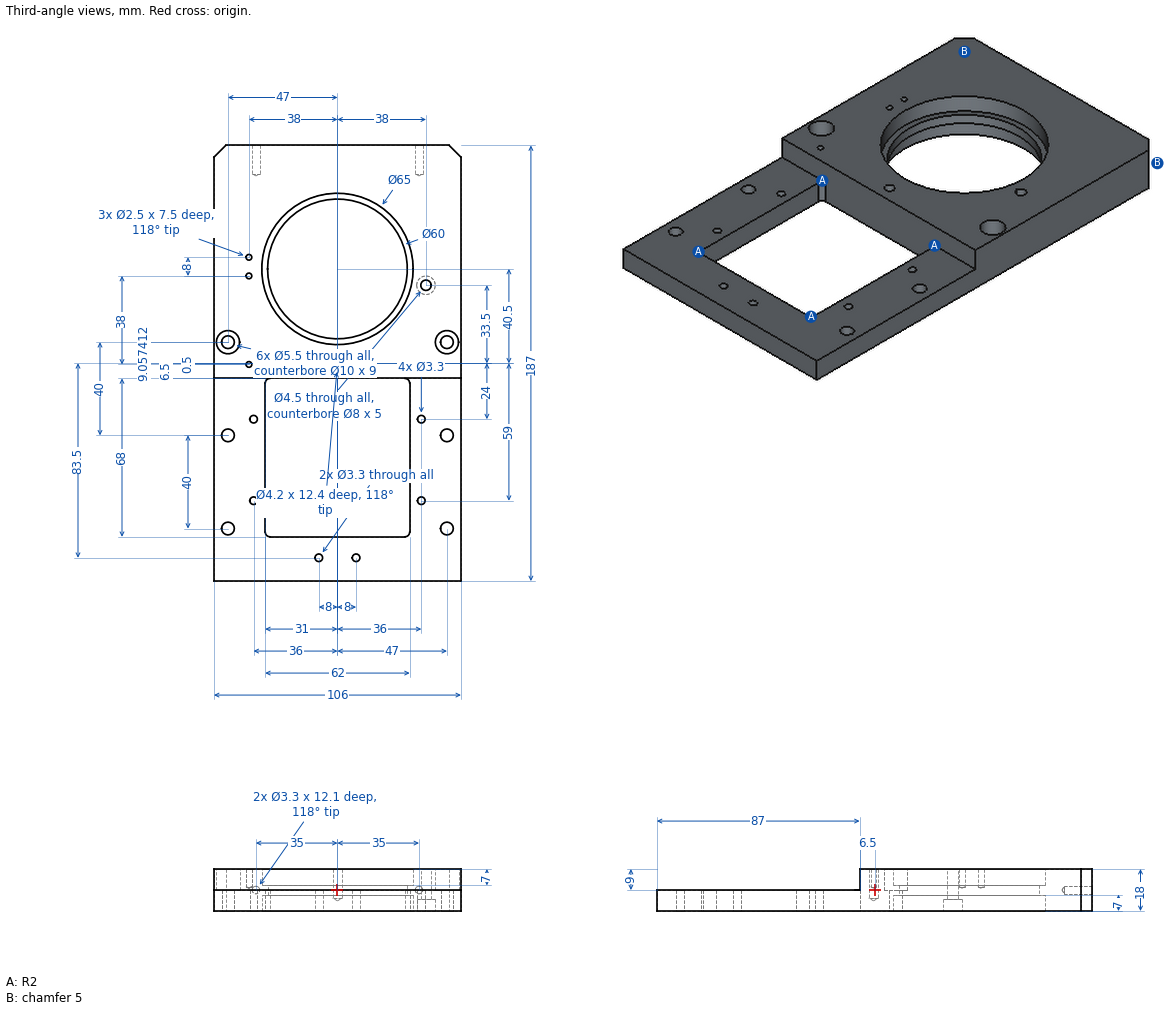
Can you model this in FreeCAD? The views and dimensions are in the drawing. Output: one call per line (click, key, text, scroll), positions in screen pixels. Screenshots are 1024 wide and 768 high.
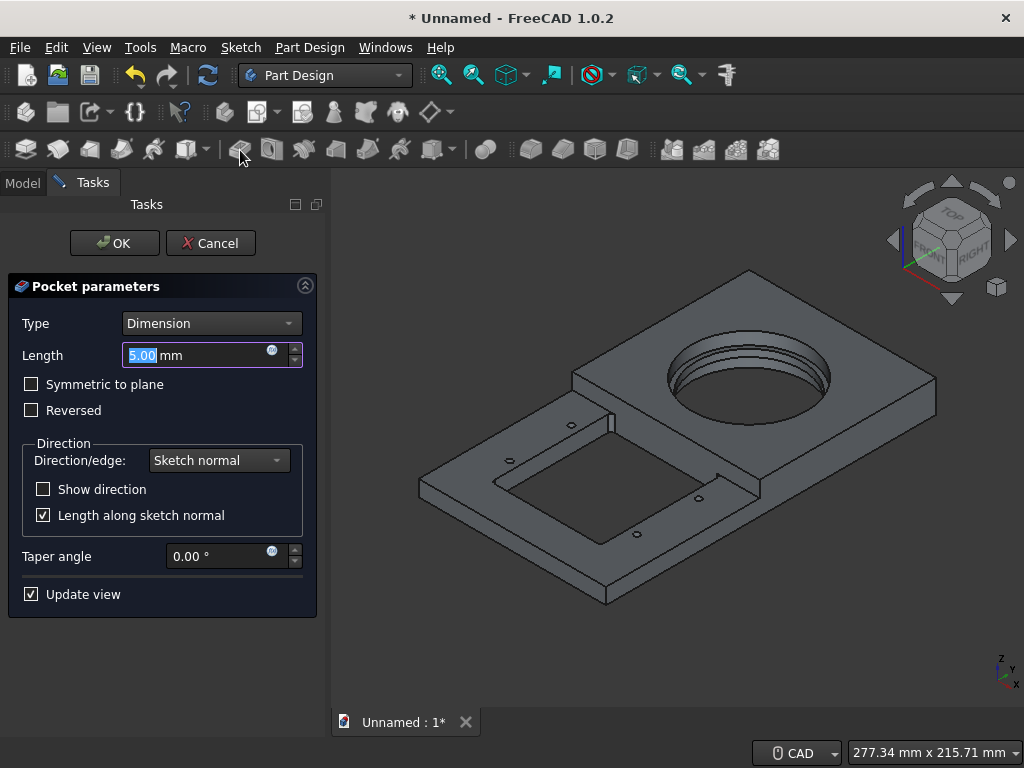
click(212, 324)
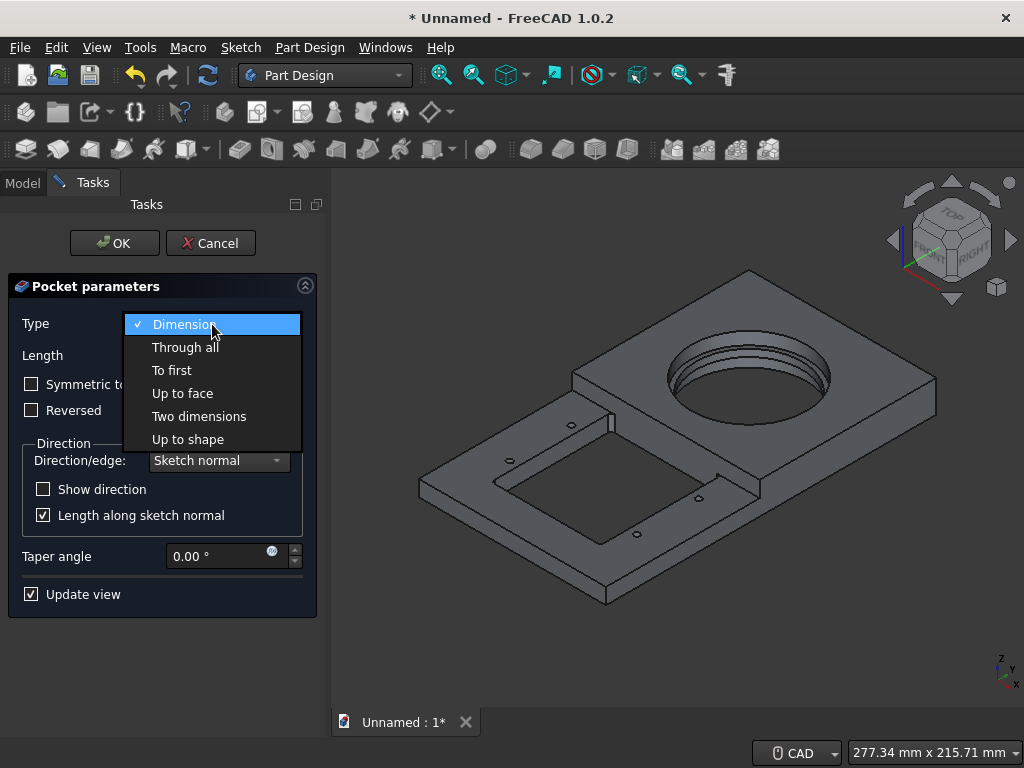
click(212, 348)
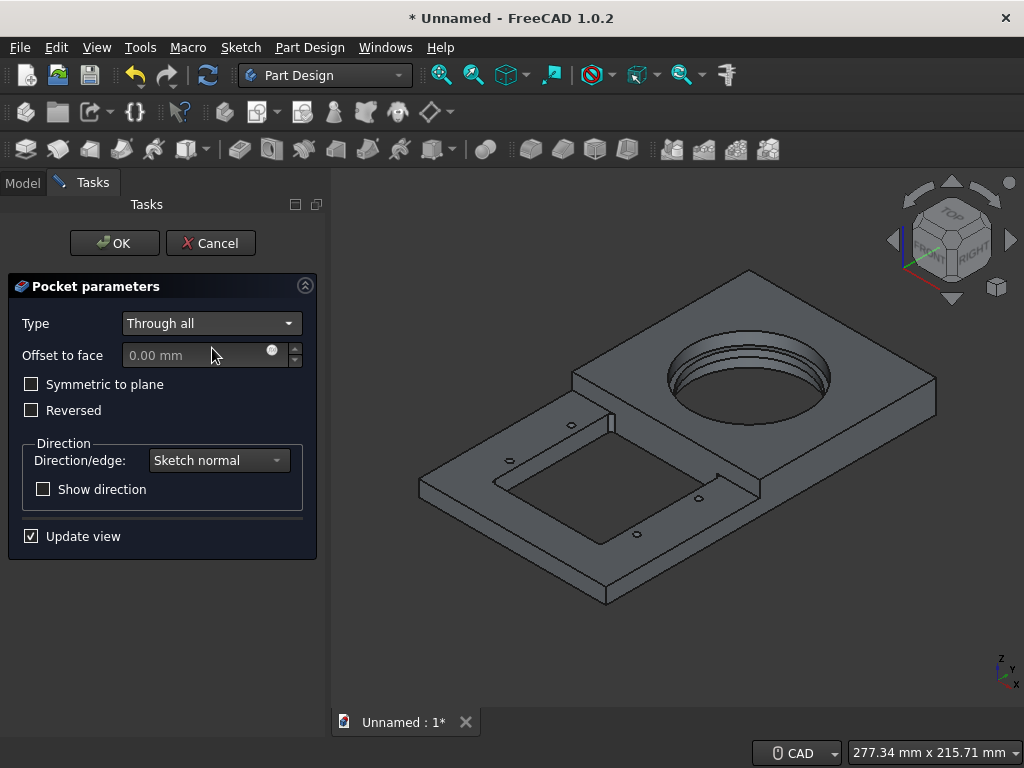
click(115, 243)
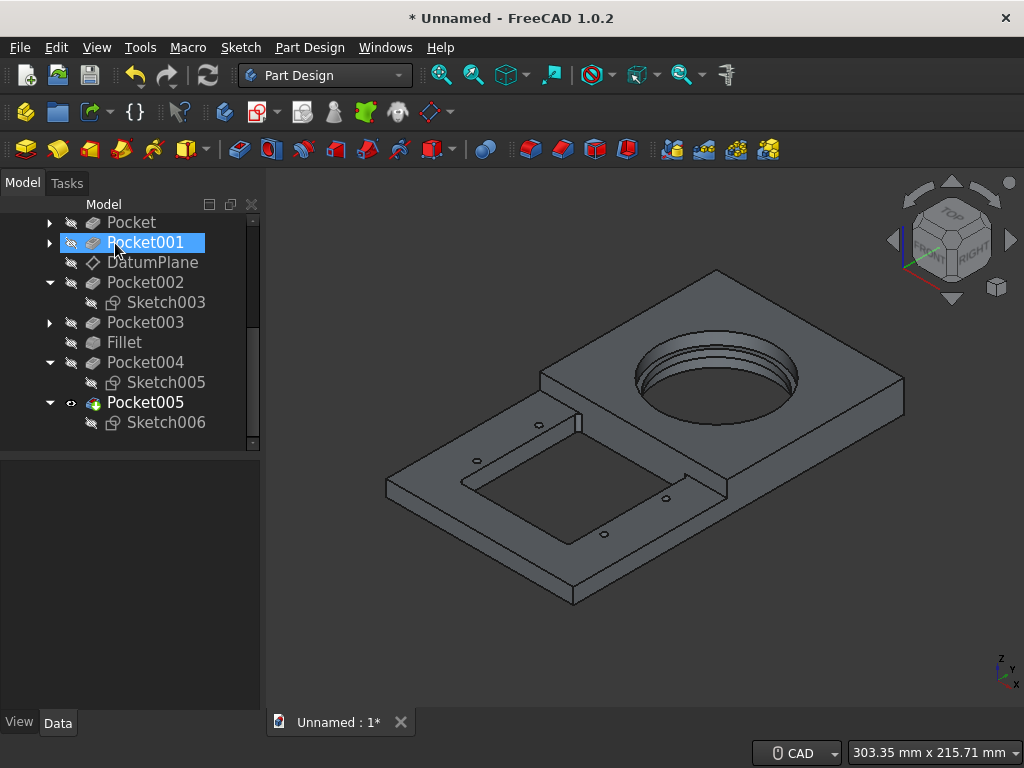
click(258, 112)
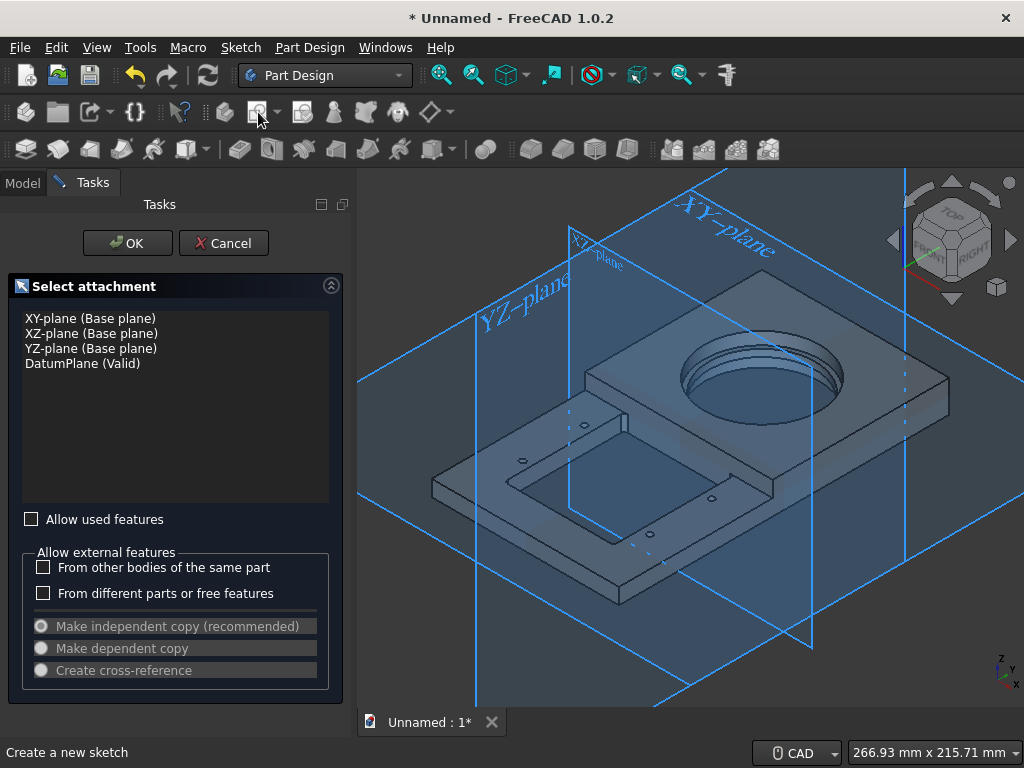
click(82, 318)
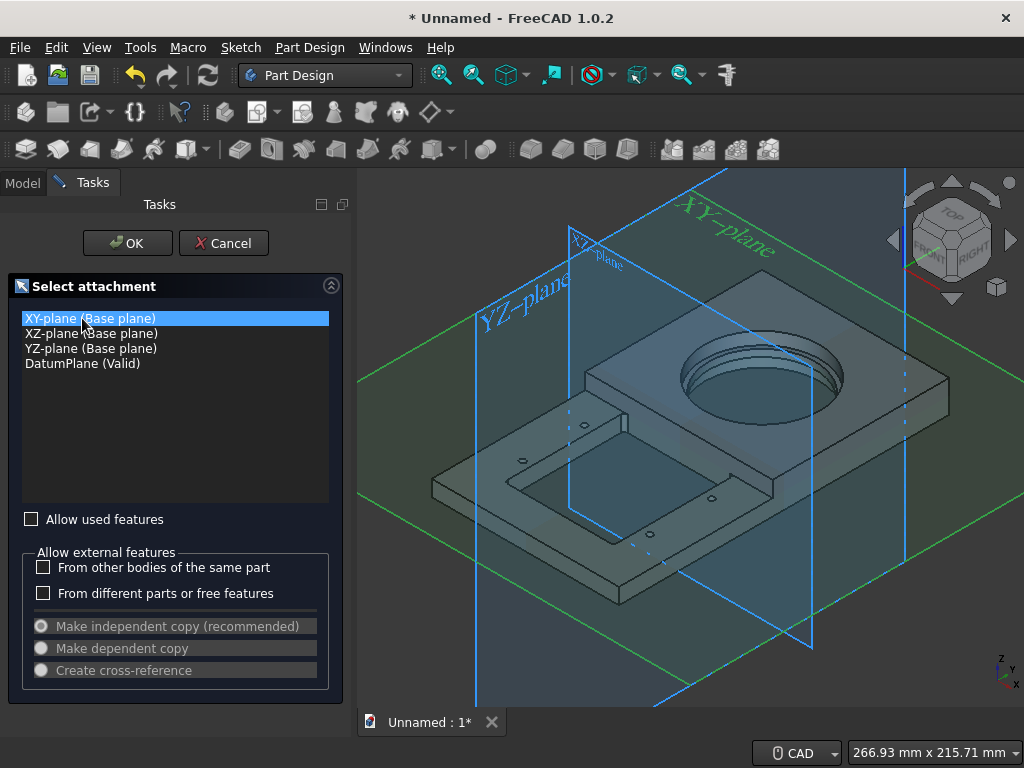
click(128, 243)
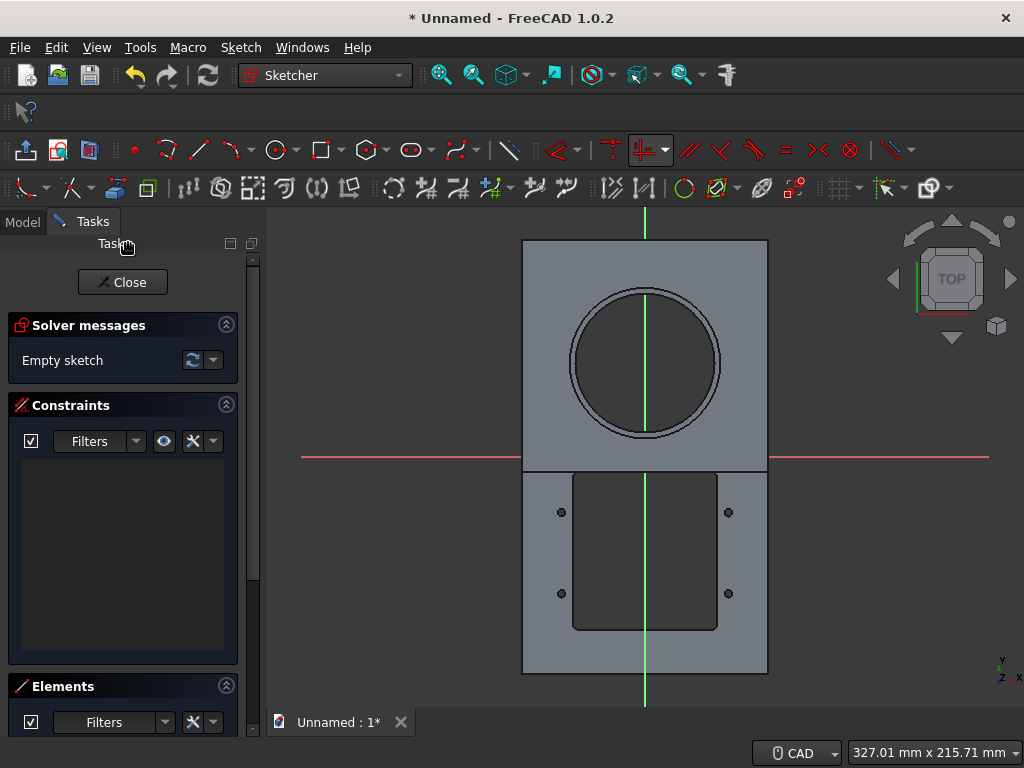
click(90, 150)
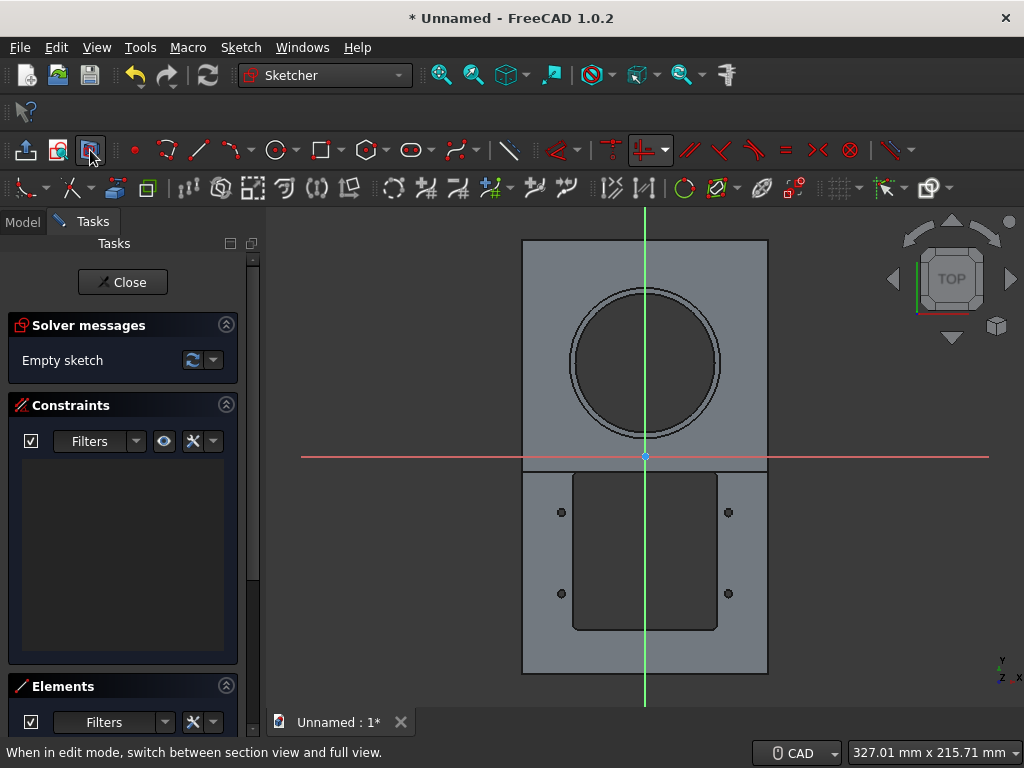
scroll(654, 675, up, 11)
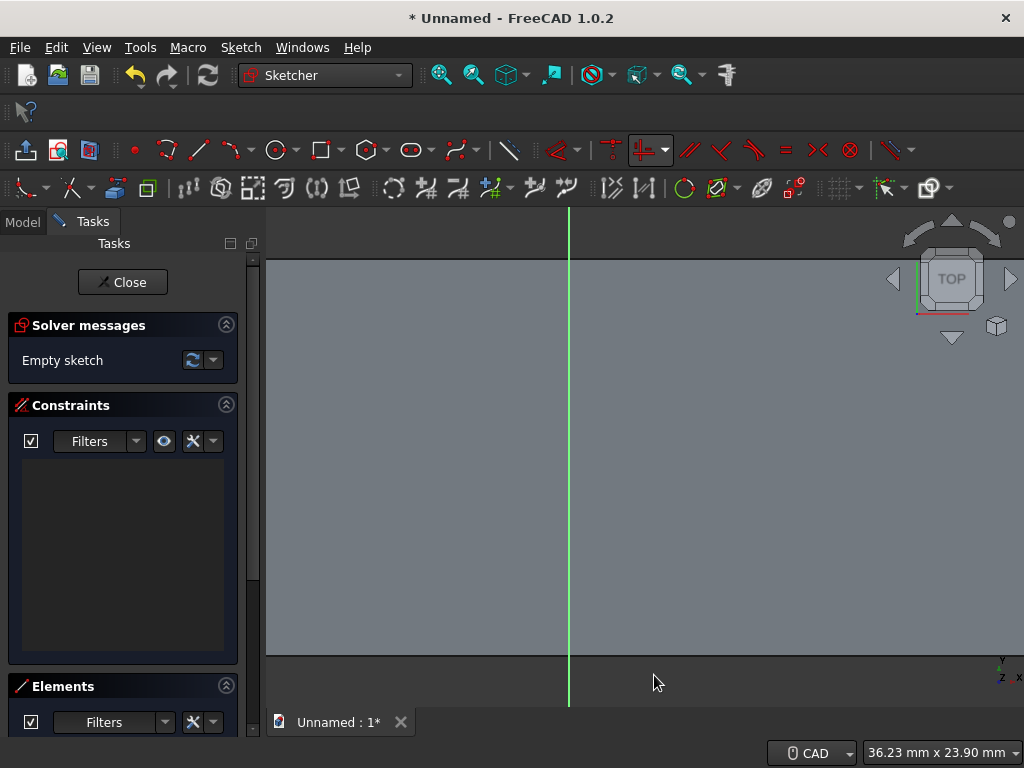
click(276, 150)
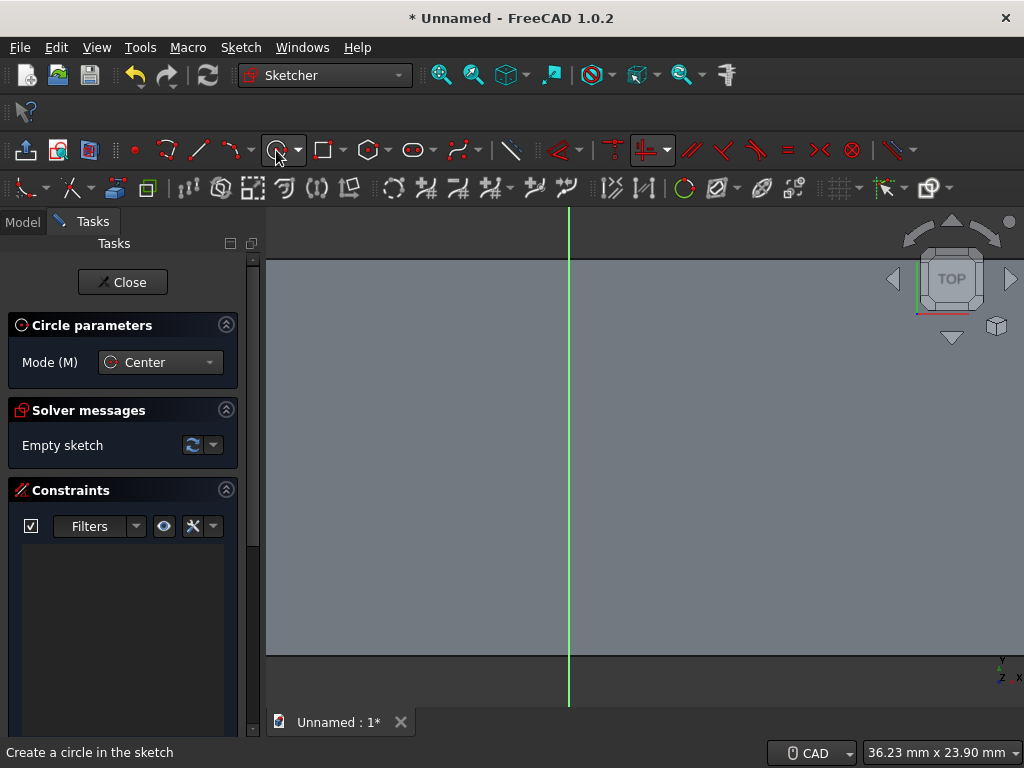
click(401, 447)
click(426, 422)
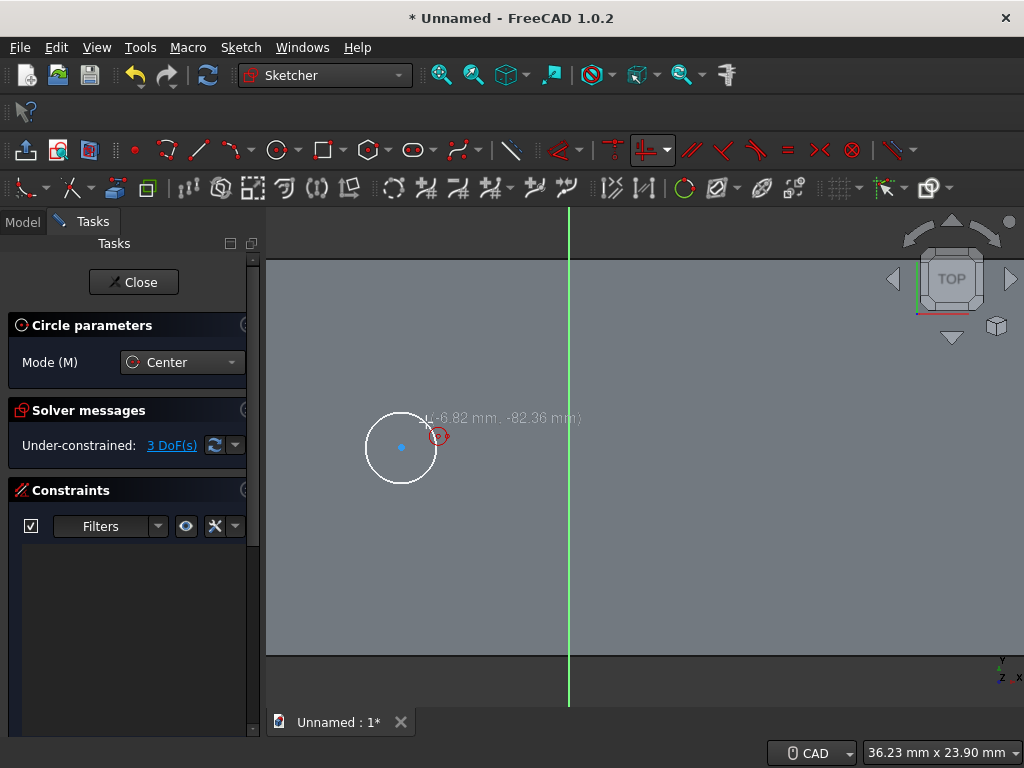
click(736, 447)
click(760, 422)
key(Escape)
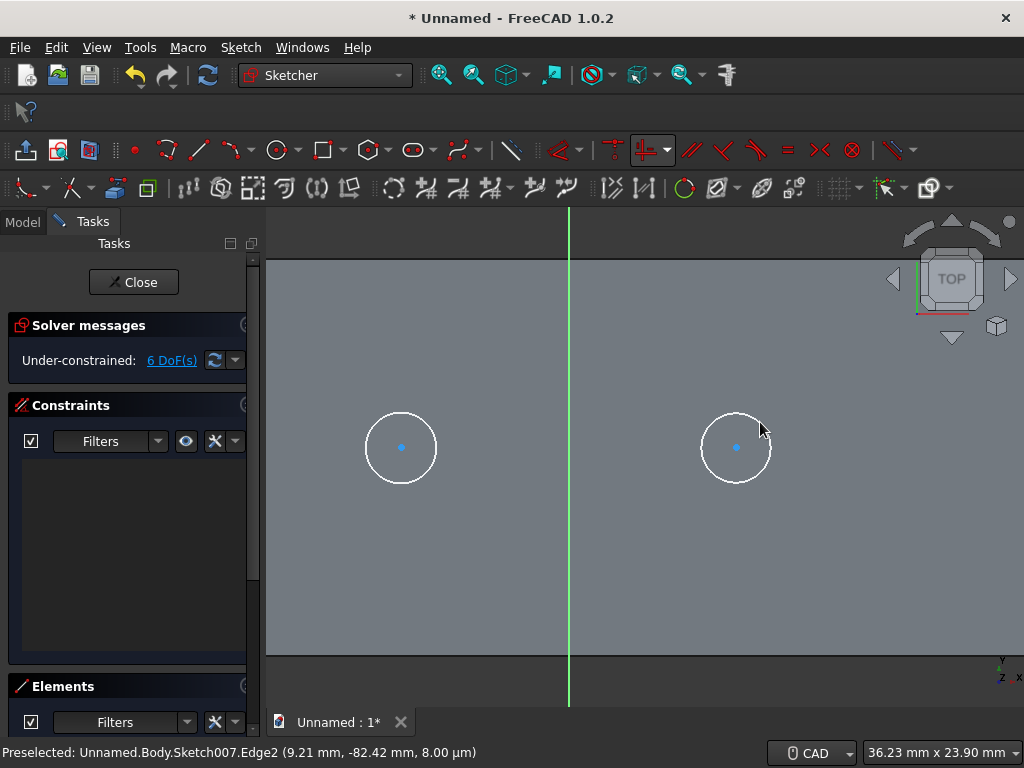
click(426, 423)